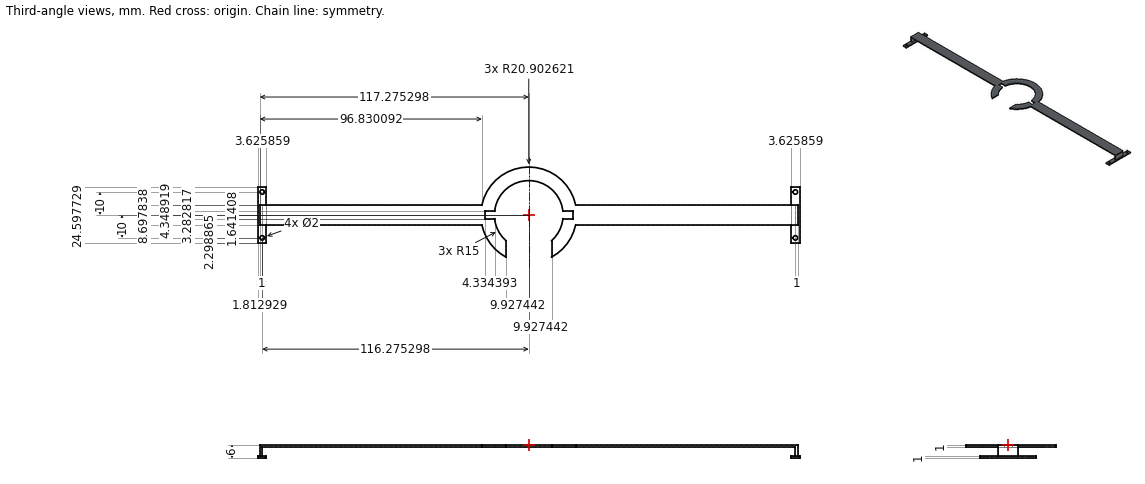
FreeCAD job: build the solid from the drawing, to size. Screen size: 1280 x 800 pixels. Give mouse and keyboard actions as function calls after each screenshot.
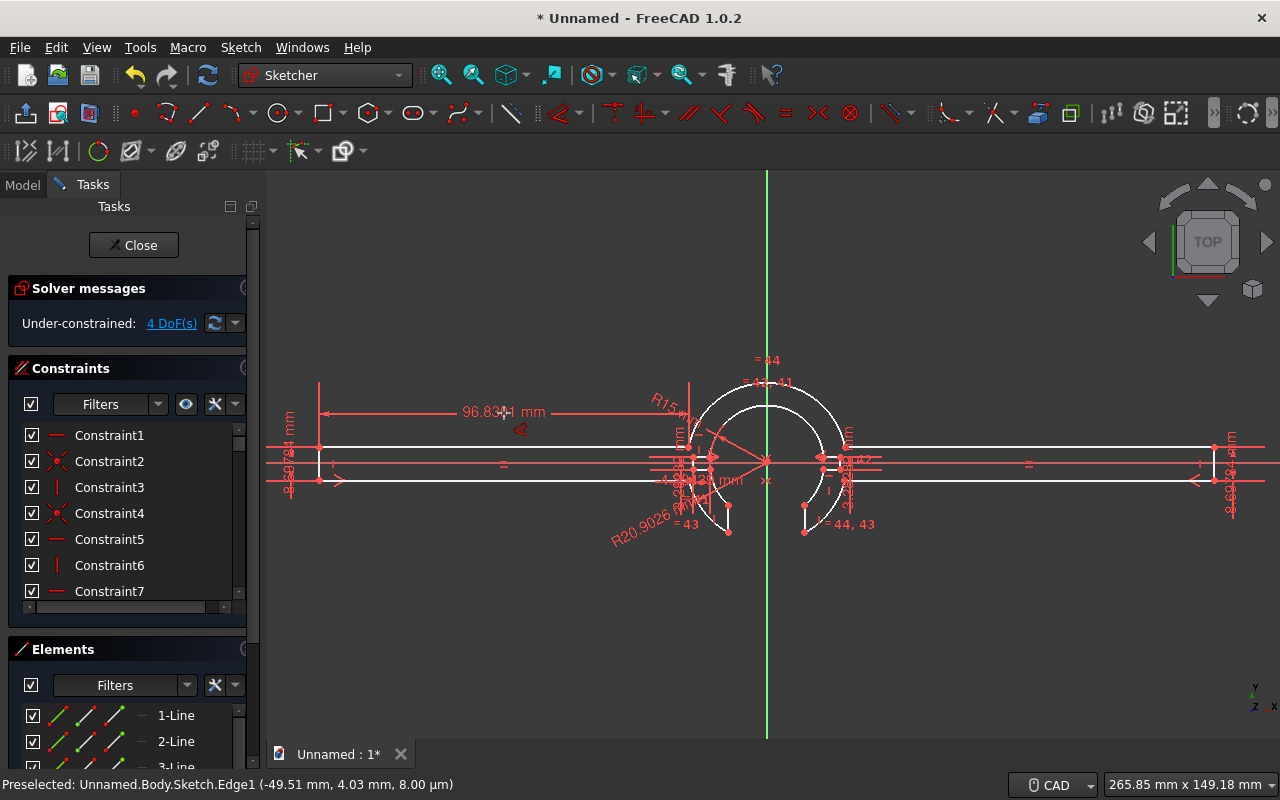
scroll(689, 447, up, 5)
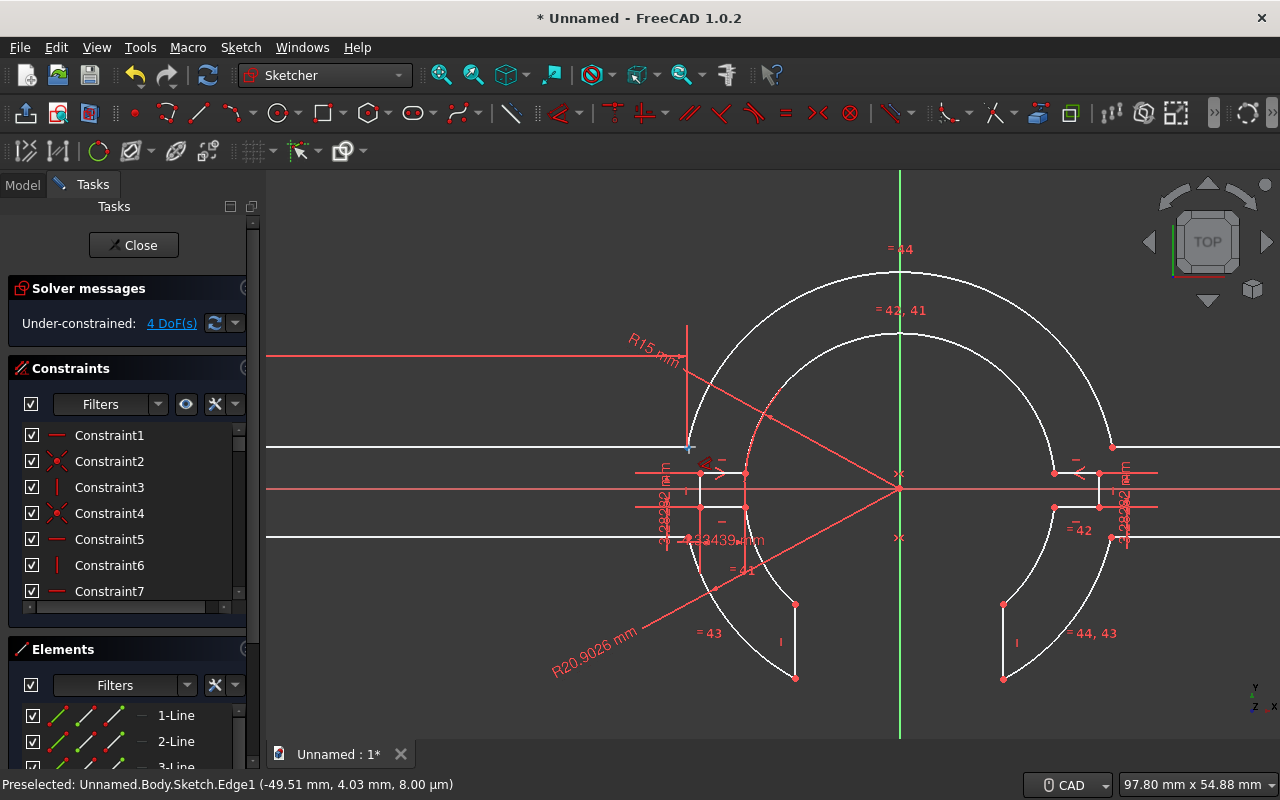
click(687, 447)
click(653, 468)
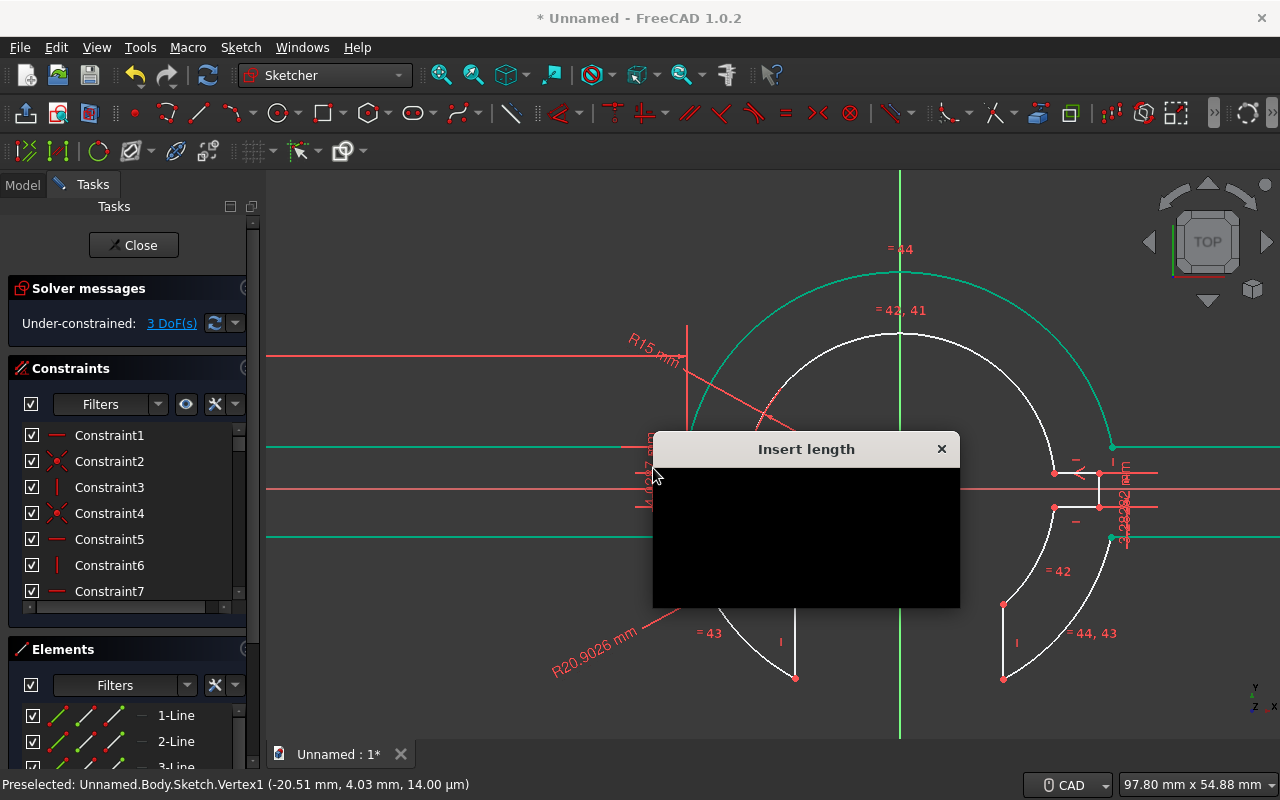
text(4.348919)
key(Return)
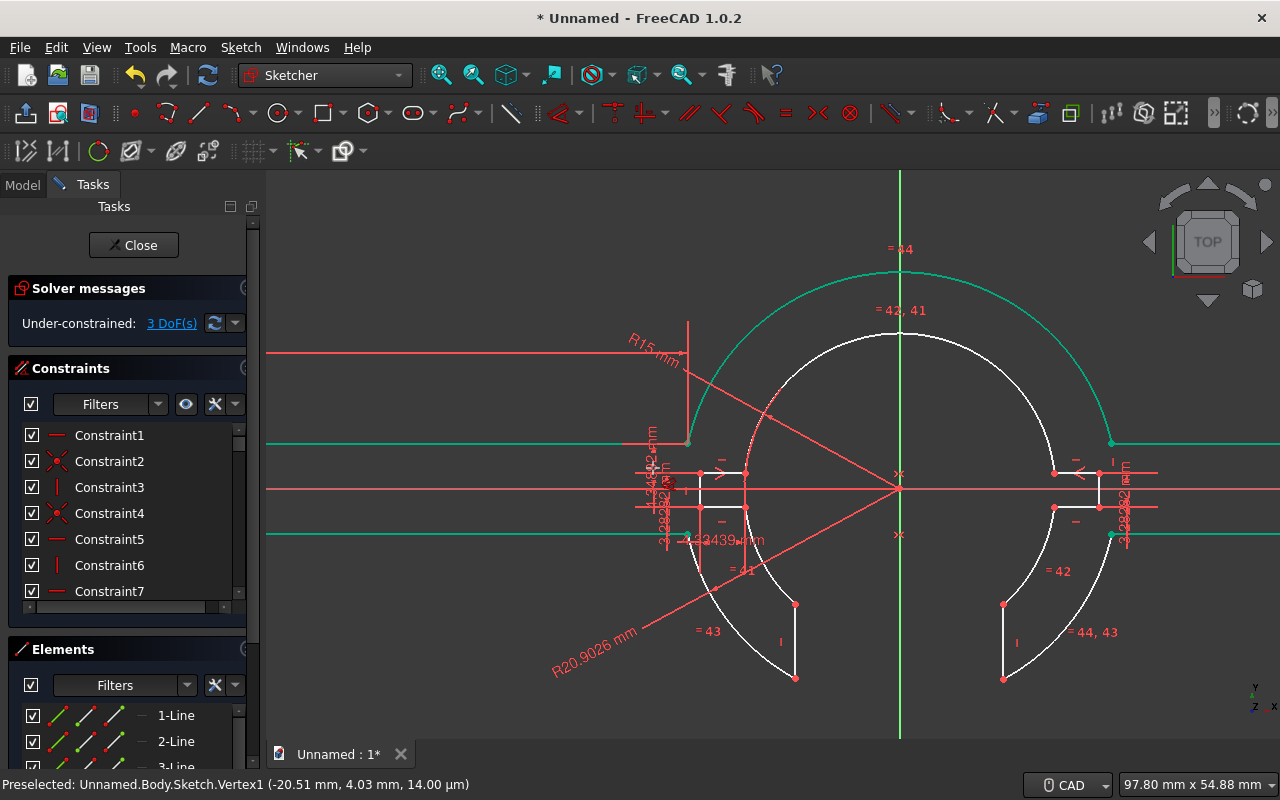
click(795, 679)
click(848, 455)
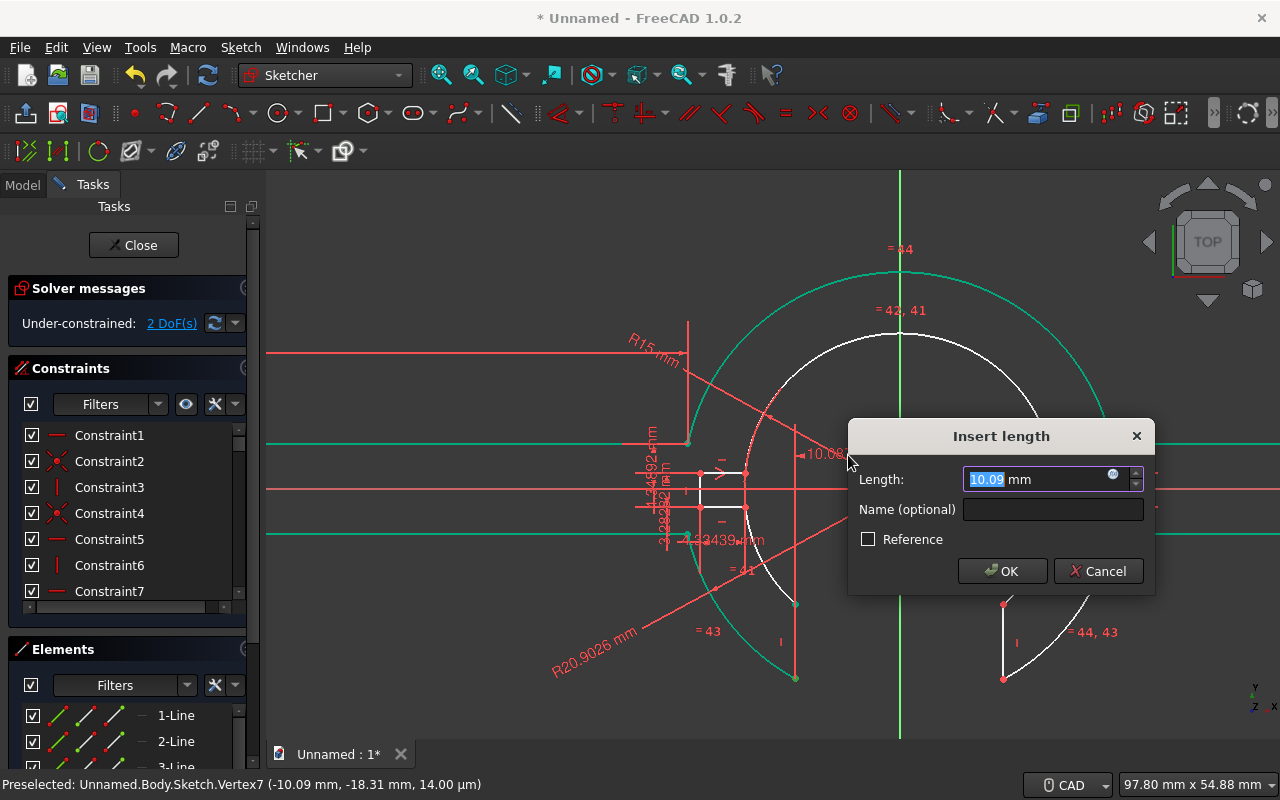
text(9.927442)
key(Return)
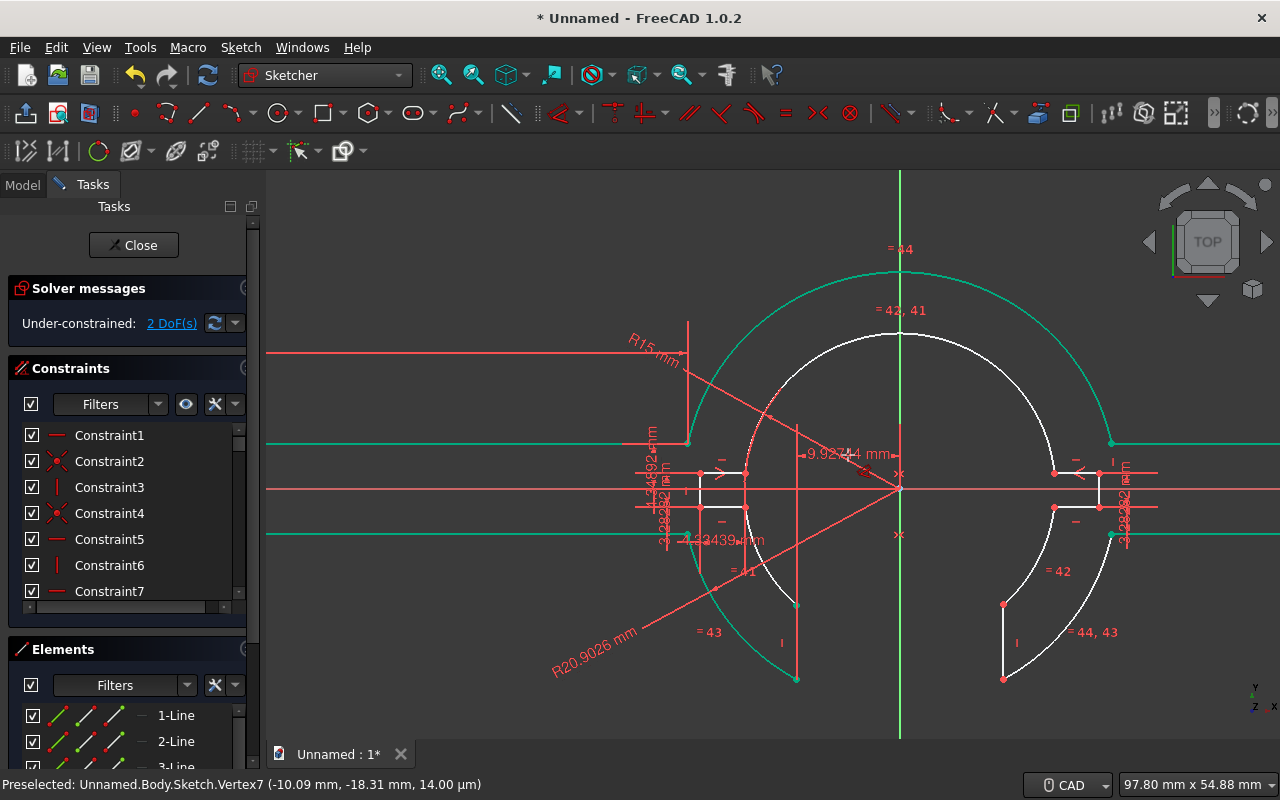
scroll(745, 507, up, 5)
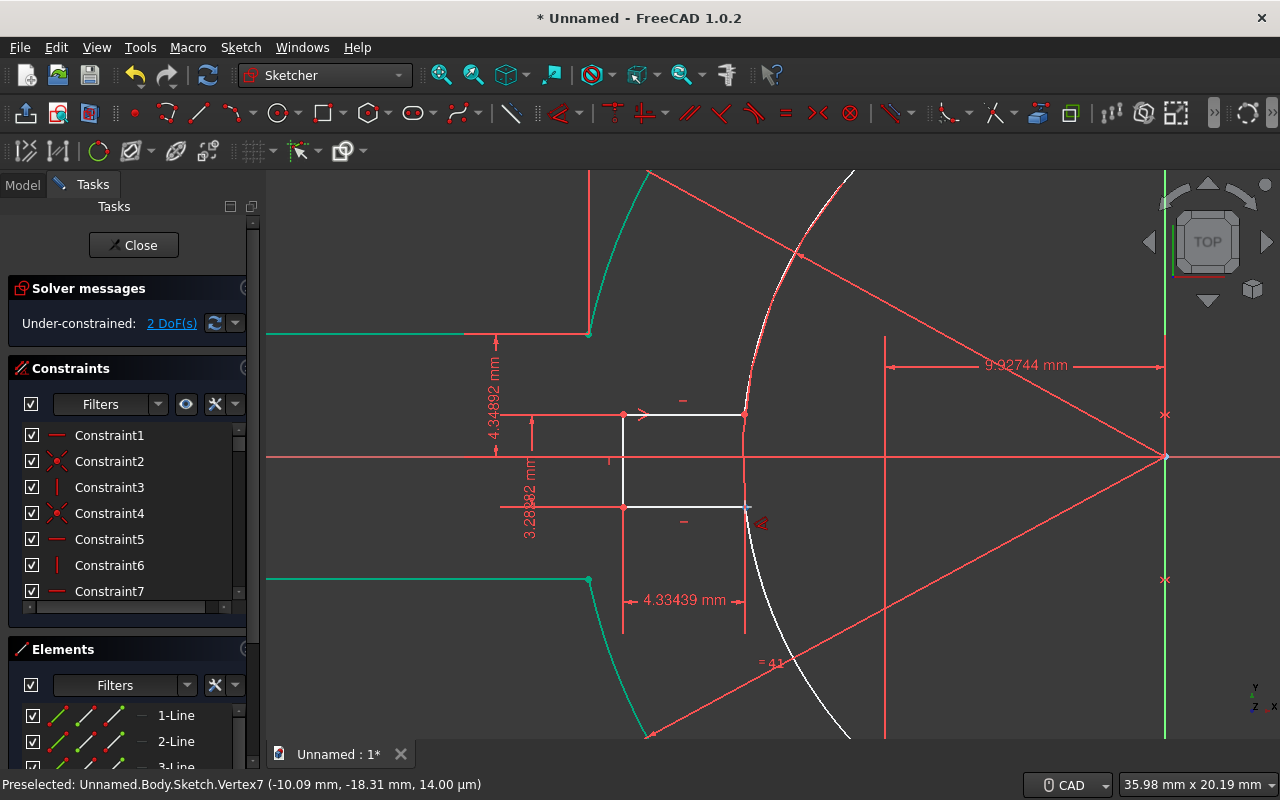
click(745, 507)
click(711, 482)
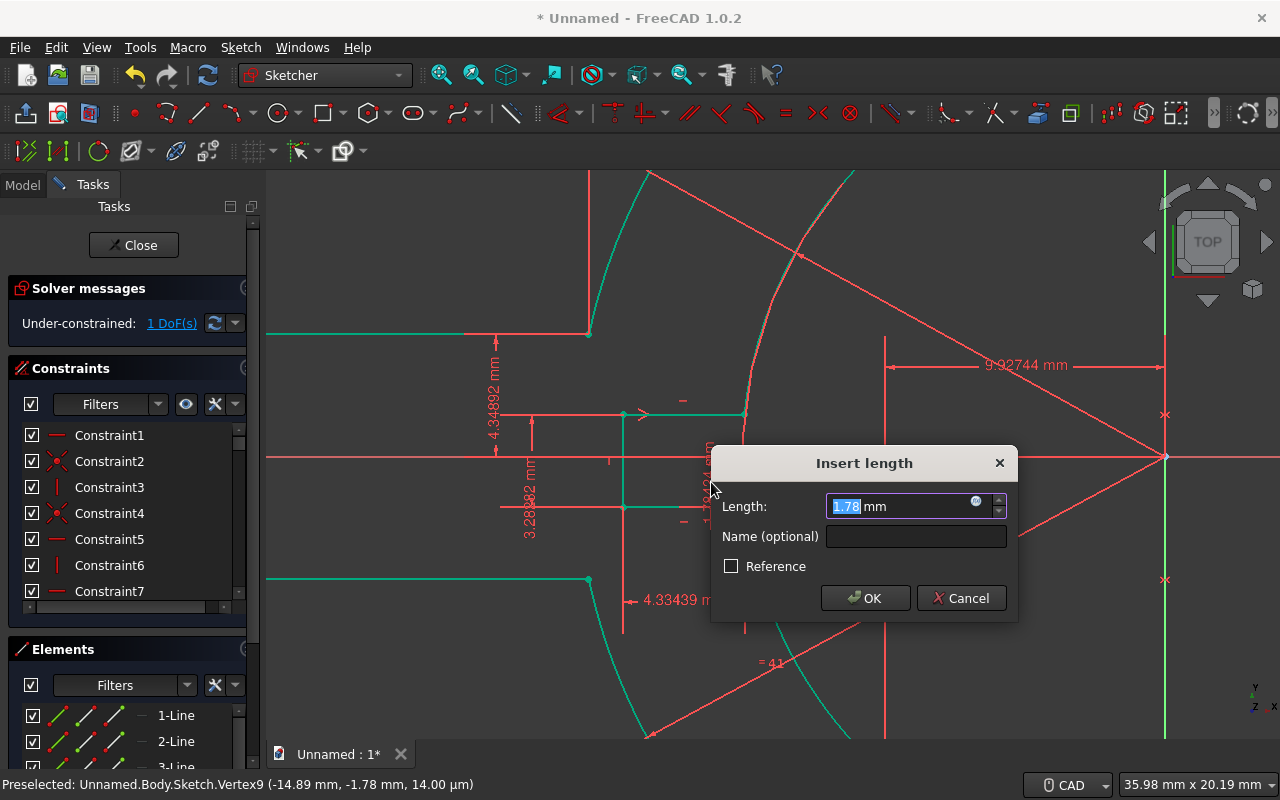
text(1.641408)
key(Return)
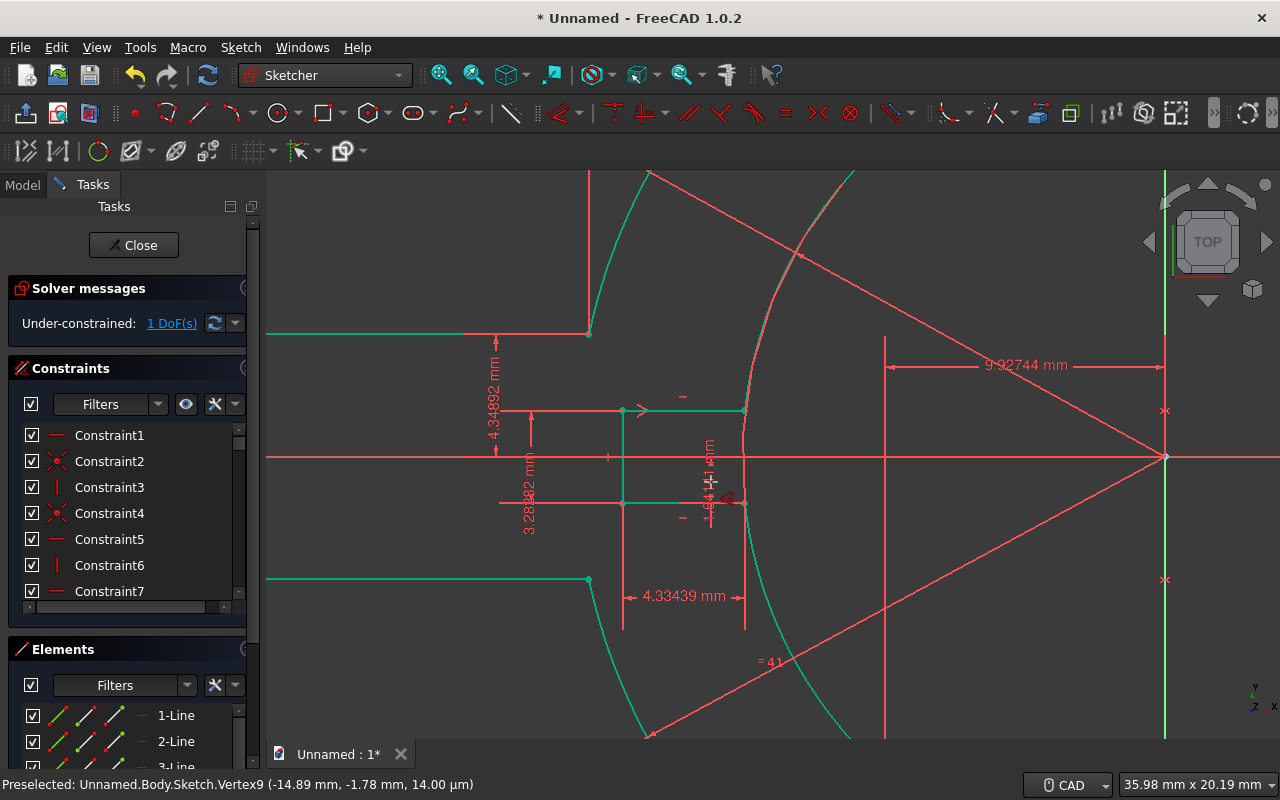
scroll(659, 458, down, 12)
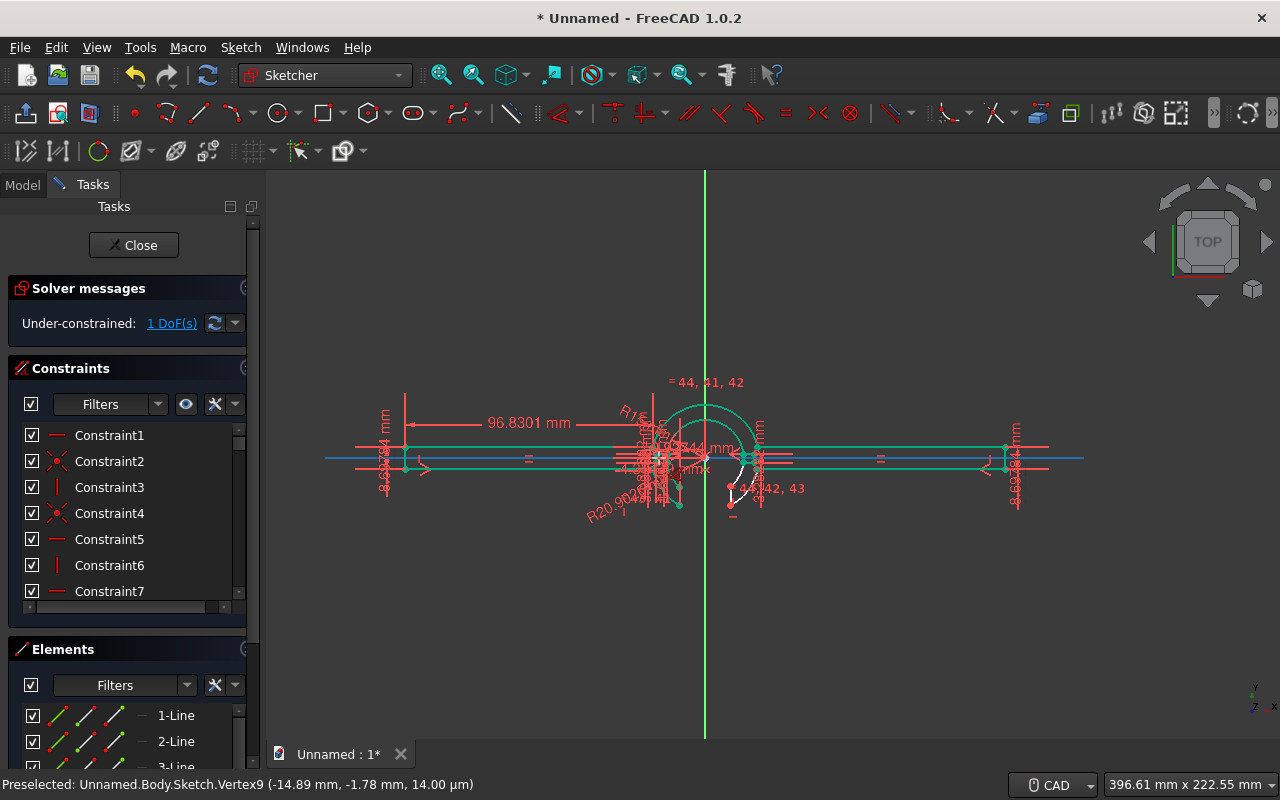
scroll(731, 487, up, 3)